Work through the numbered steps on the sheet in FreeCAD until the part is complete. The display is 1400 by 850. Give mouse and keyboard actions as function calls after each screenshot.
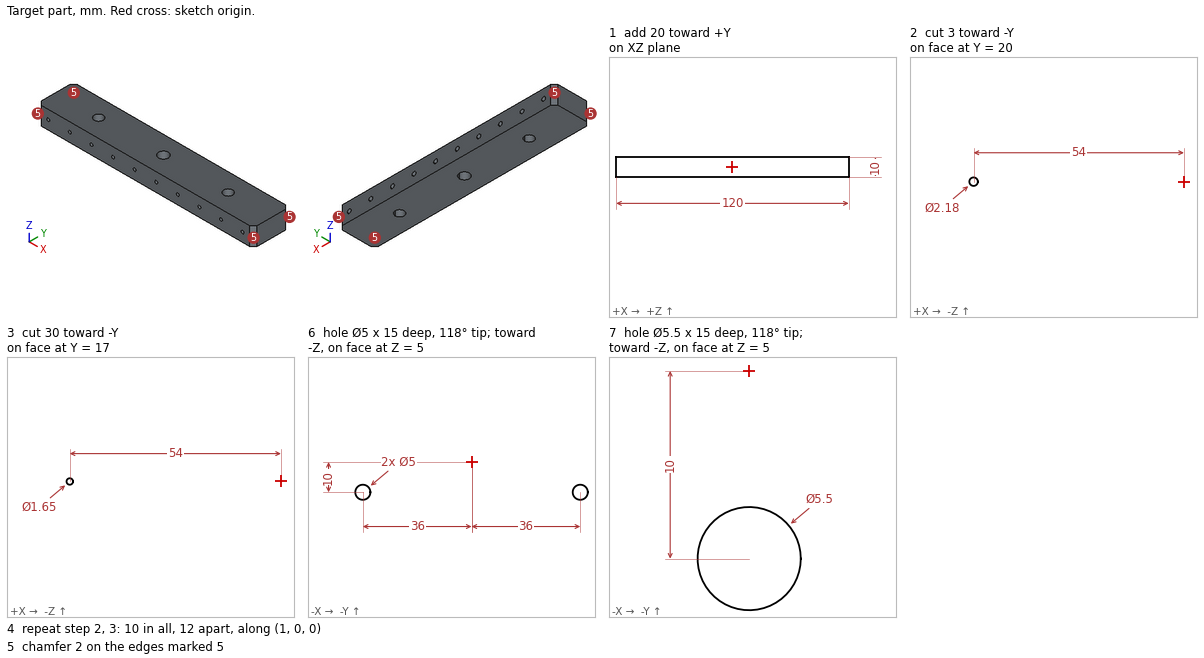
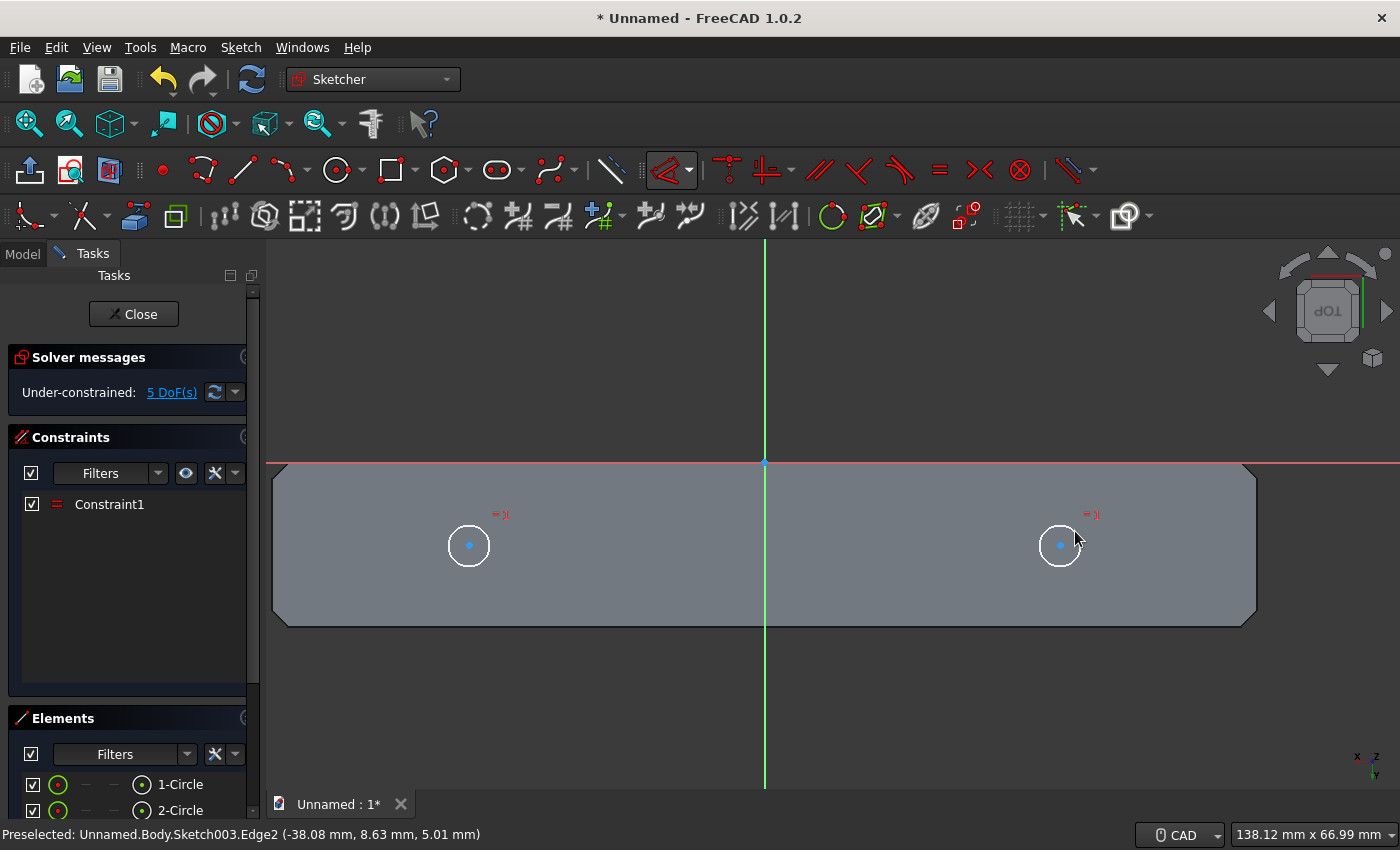
click(469, 546)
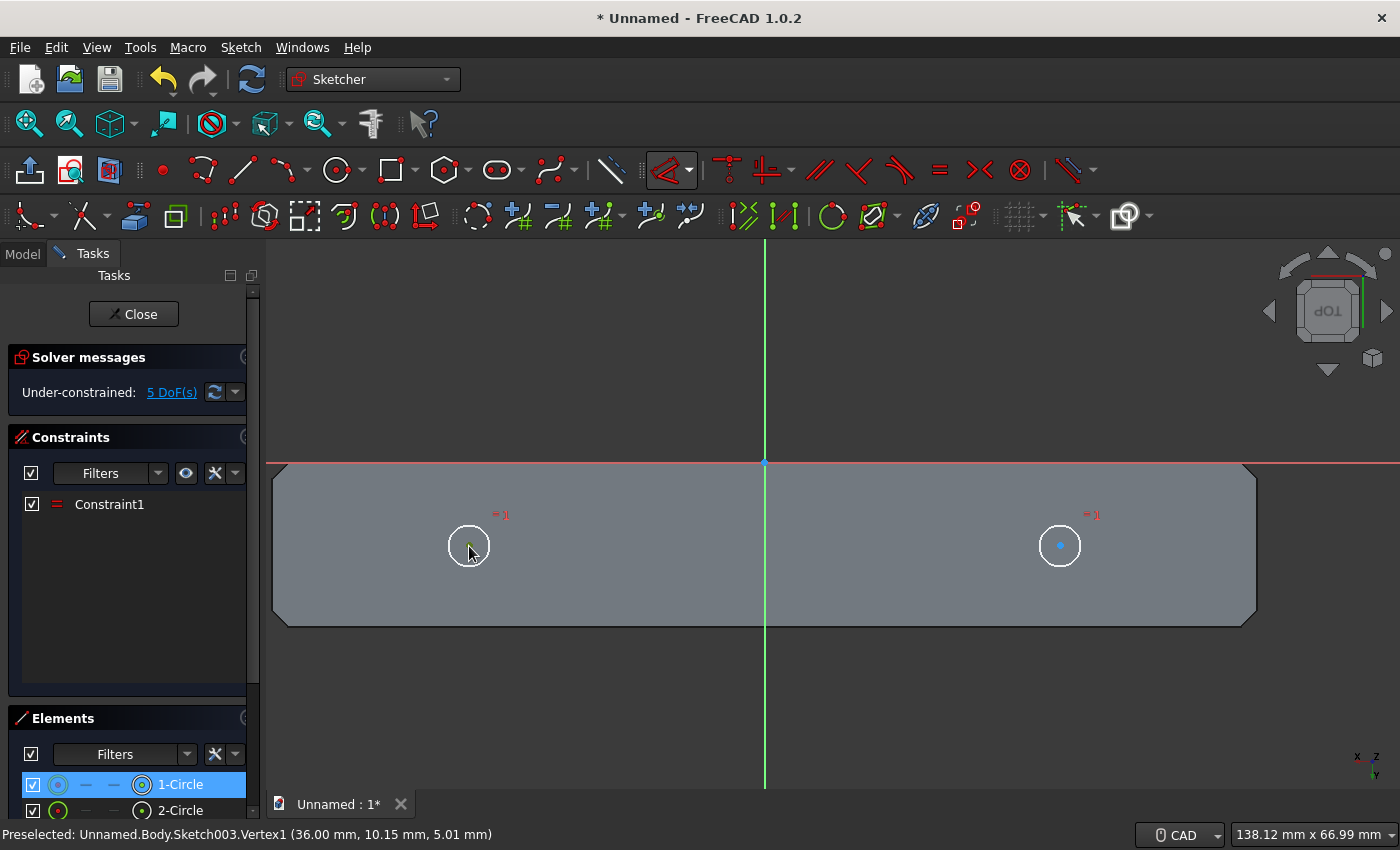
click(1060, 546)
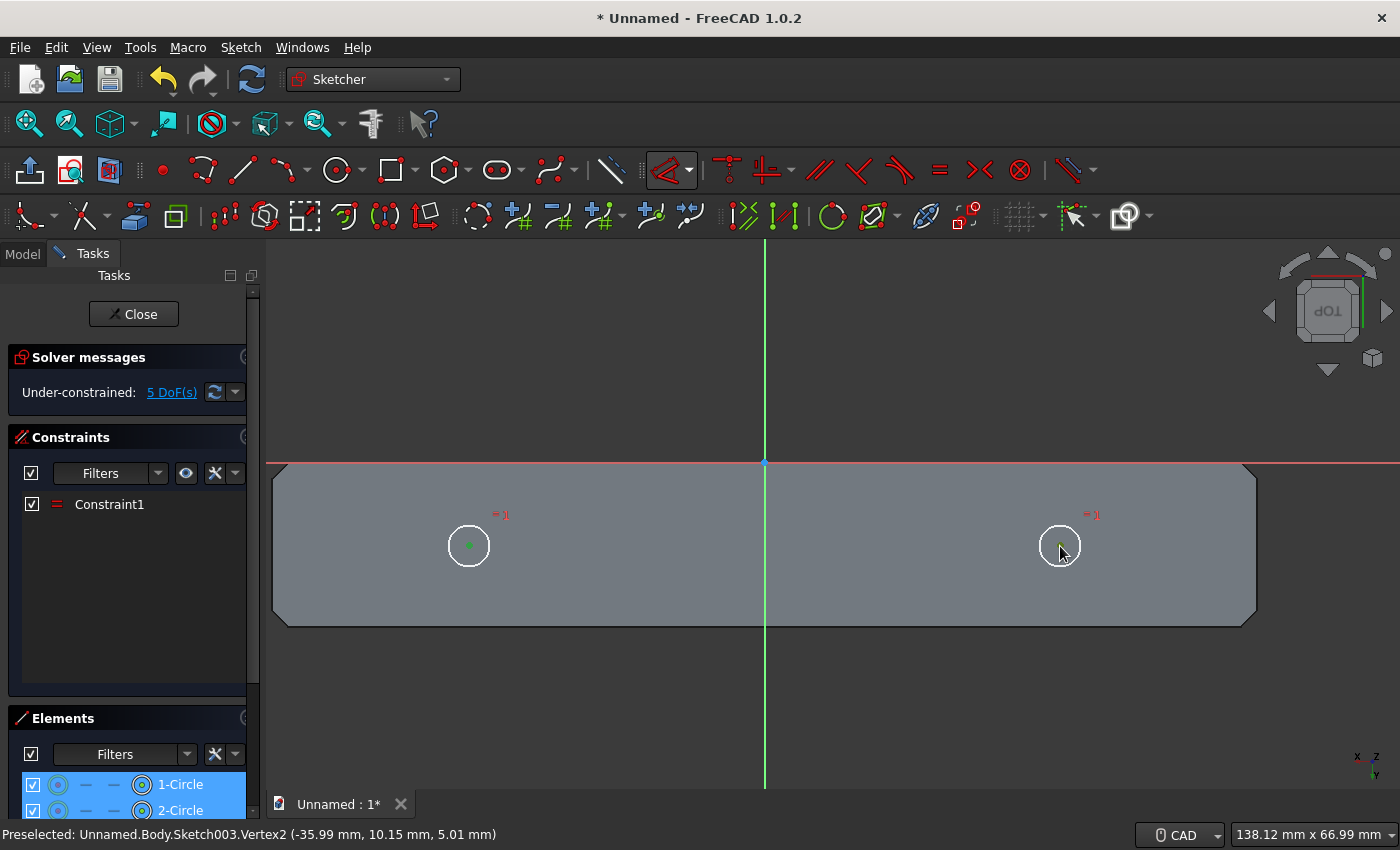
key(h)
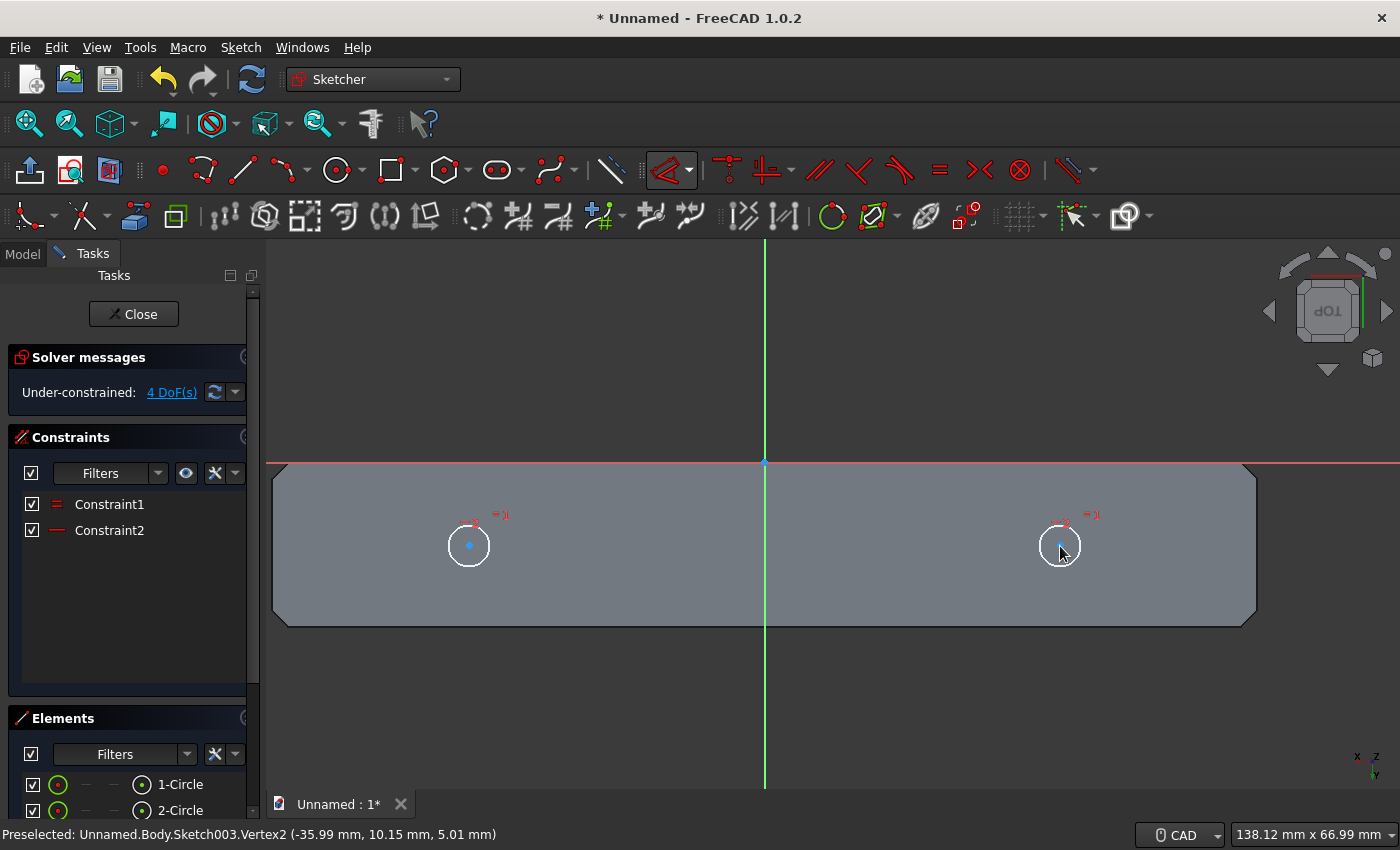
click(483, 531)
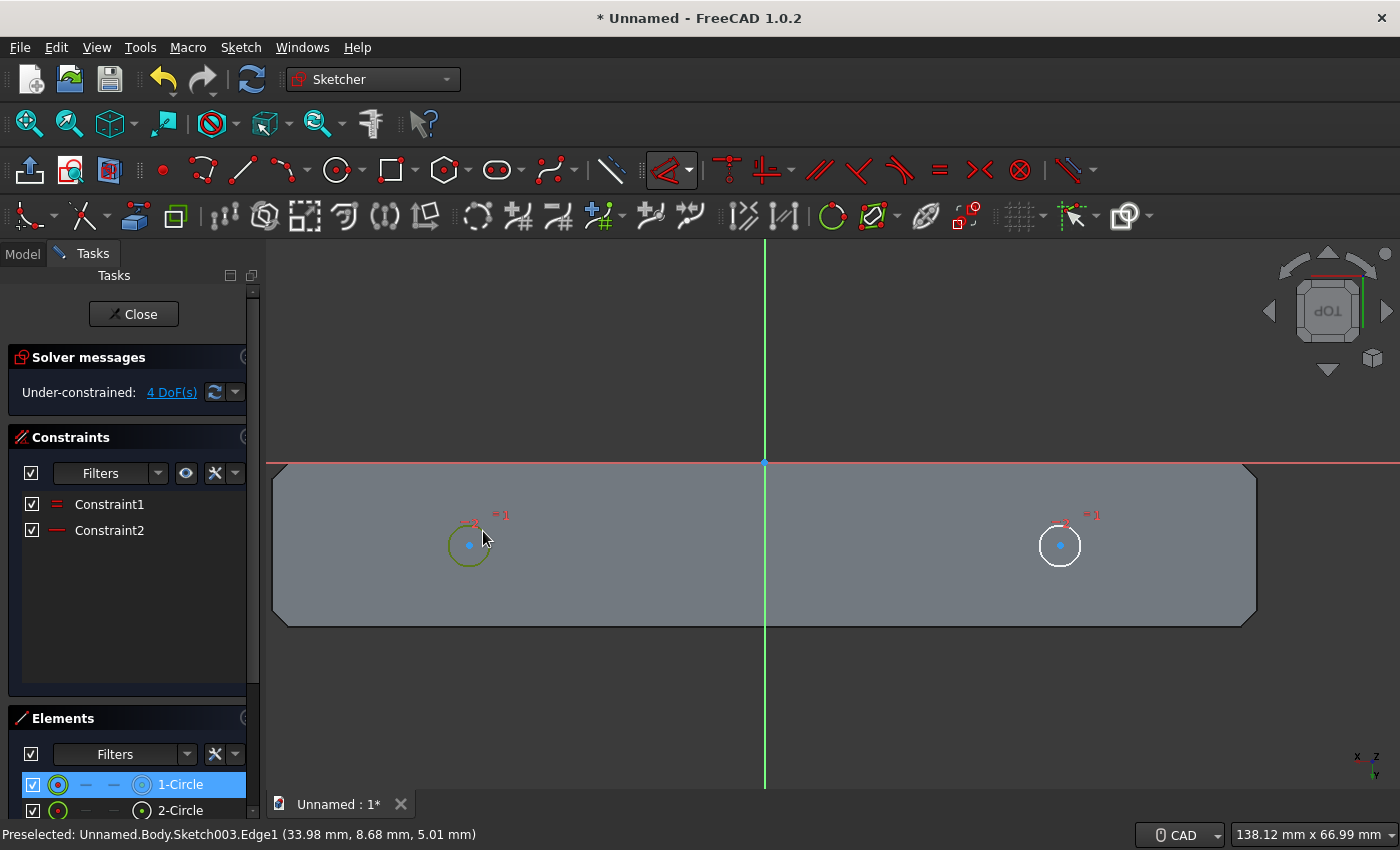
click(692, 170)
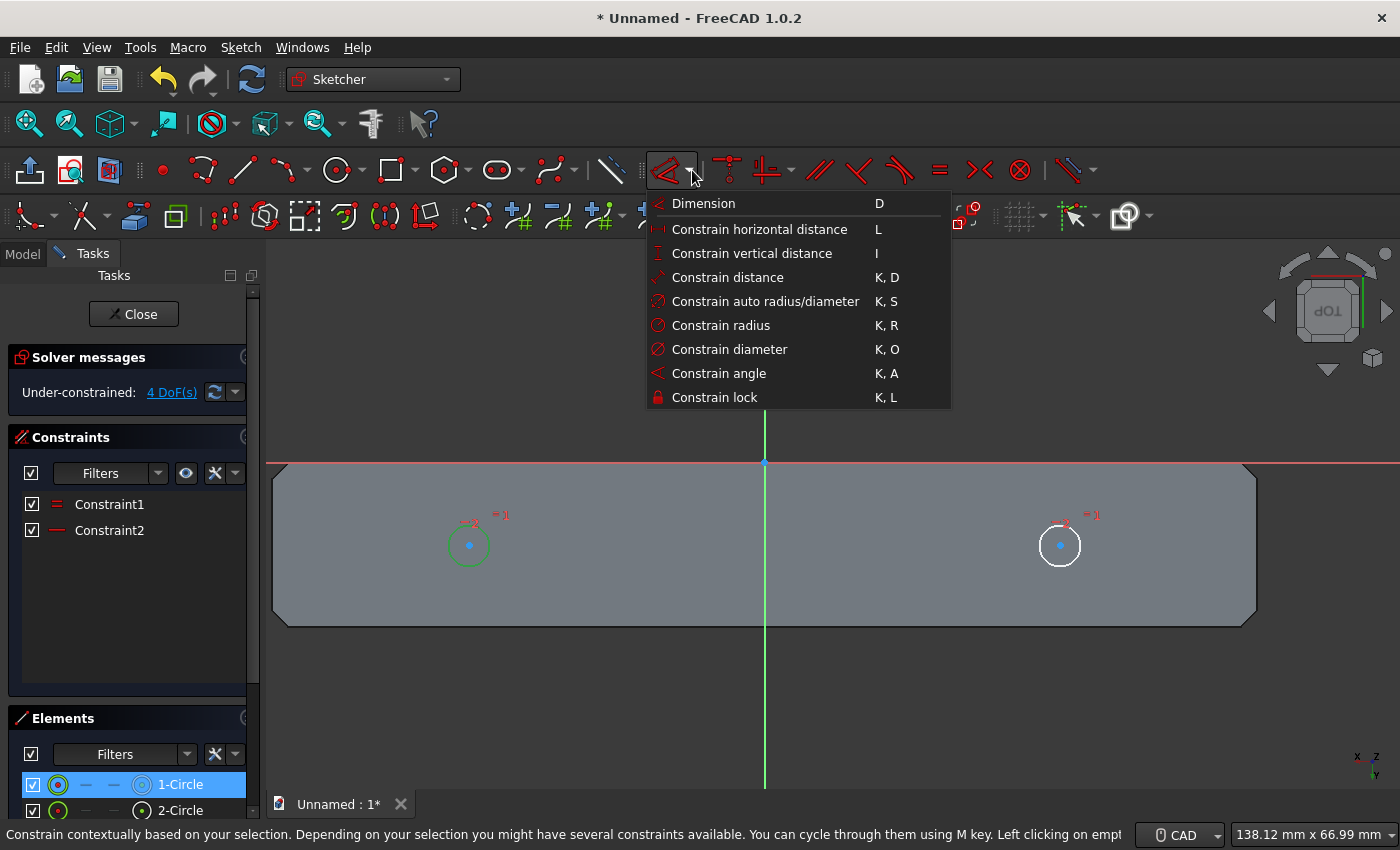
click(799, 349)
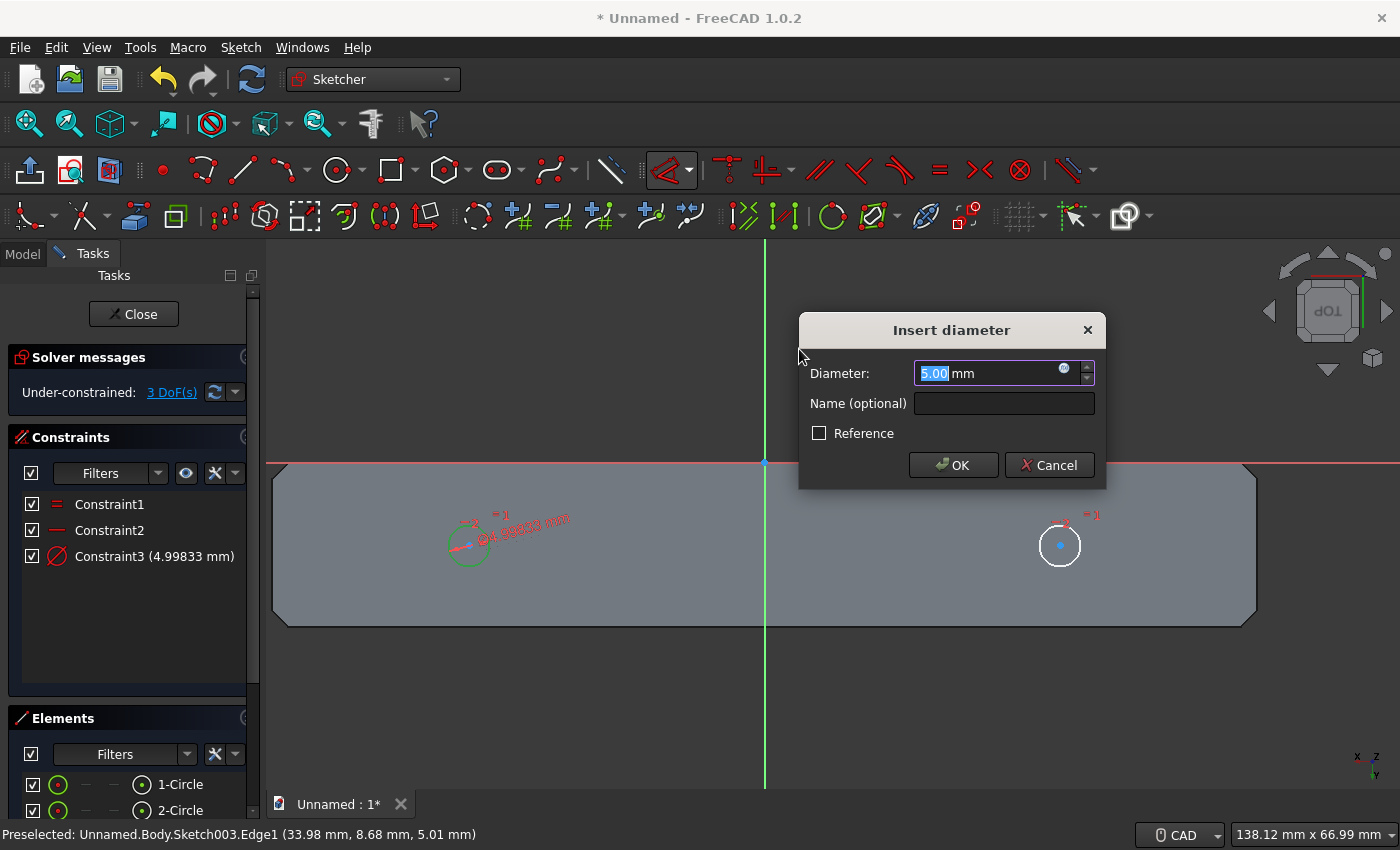
text(5)
key(Return)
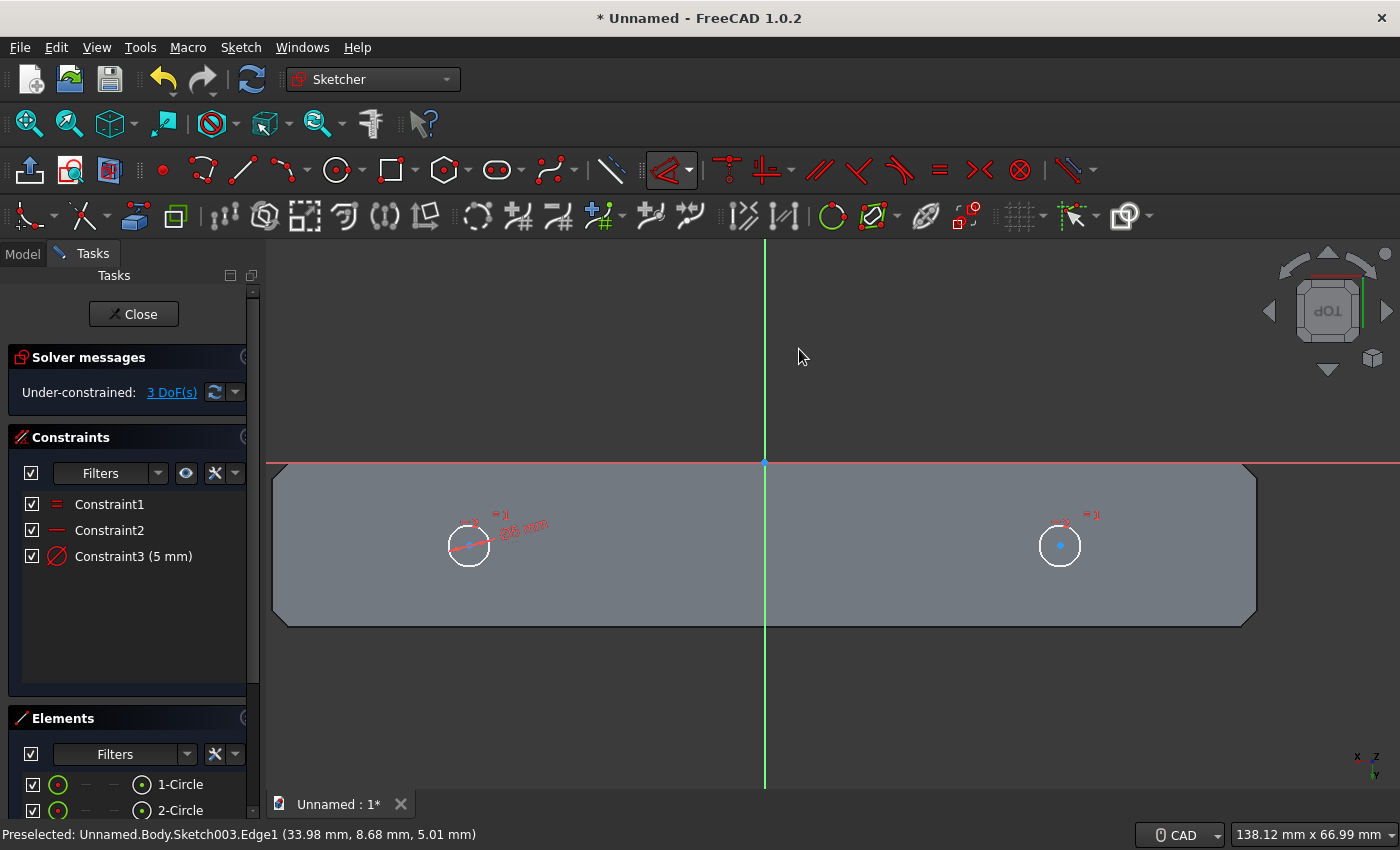
click(469, 546)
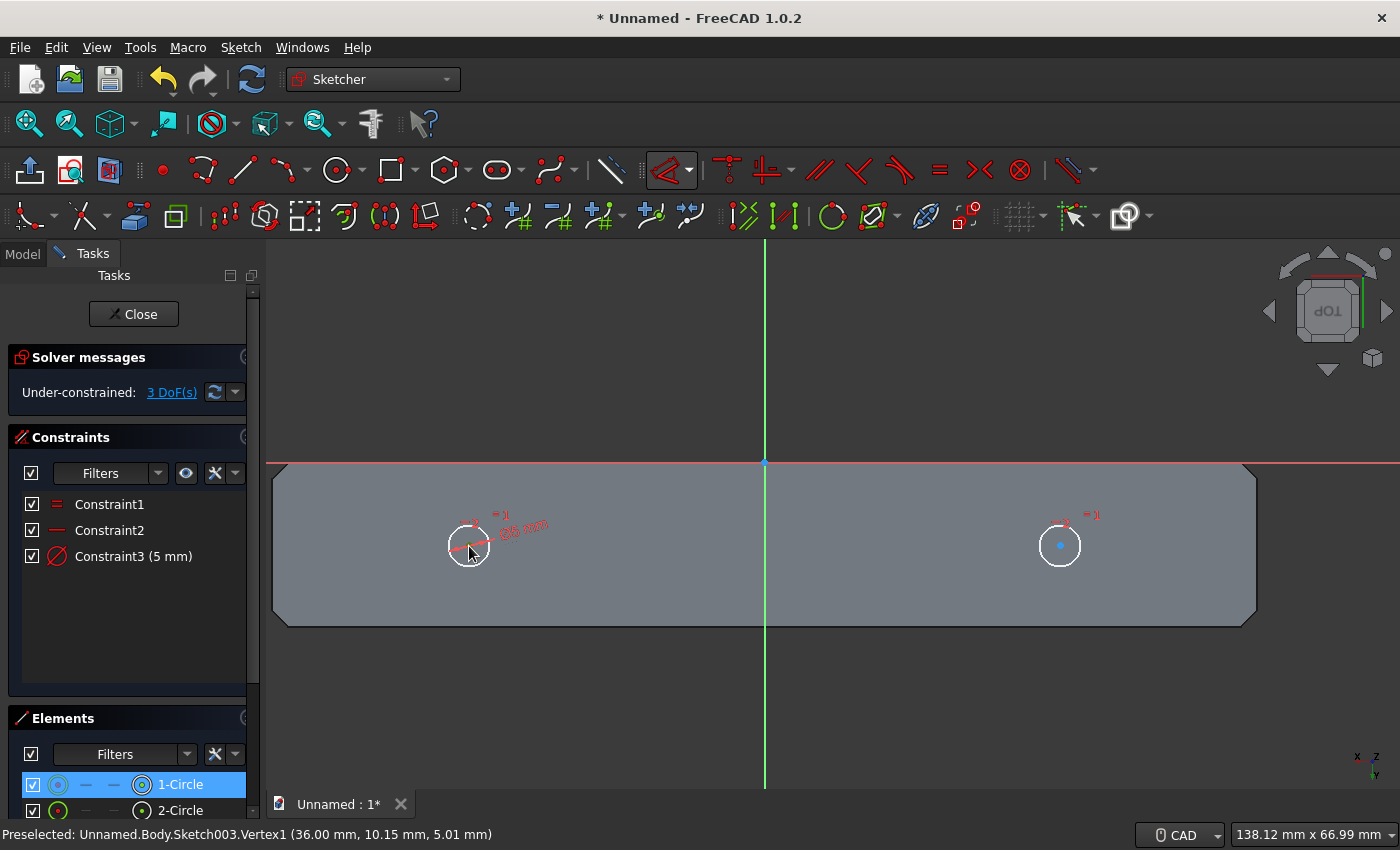
key(l)